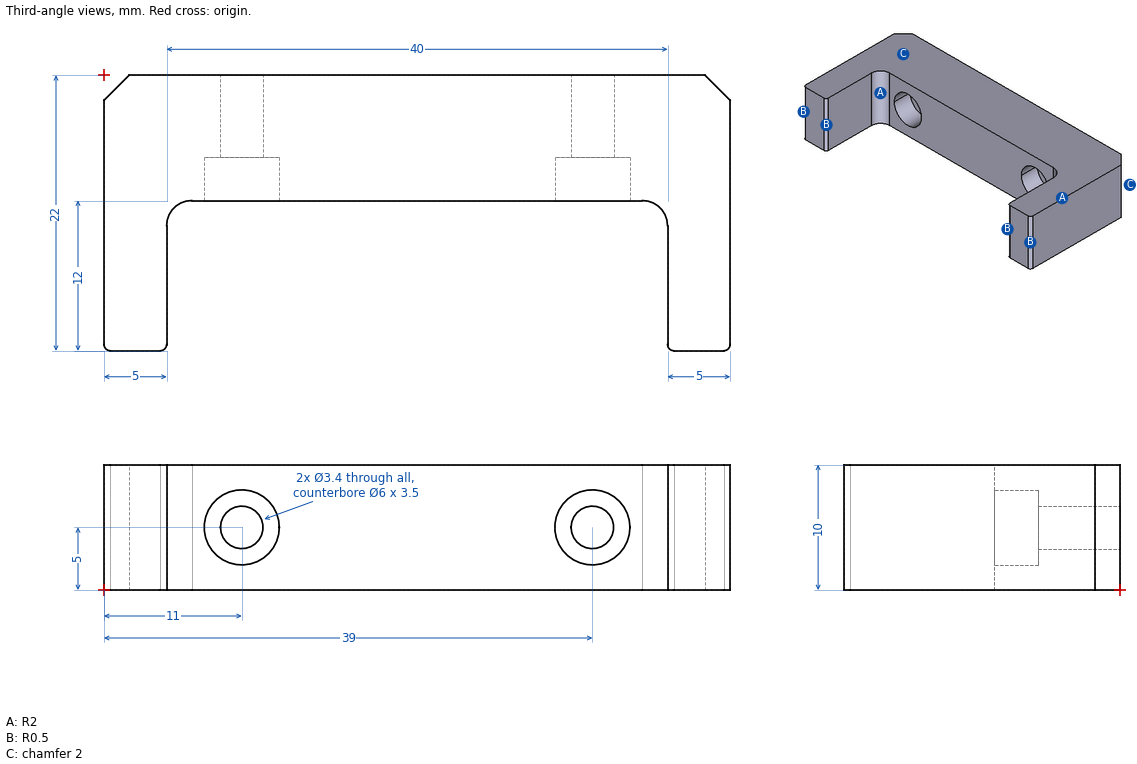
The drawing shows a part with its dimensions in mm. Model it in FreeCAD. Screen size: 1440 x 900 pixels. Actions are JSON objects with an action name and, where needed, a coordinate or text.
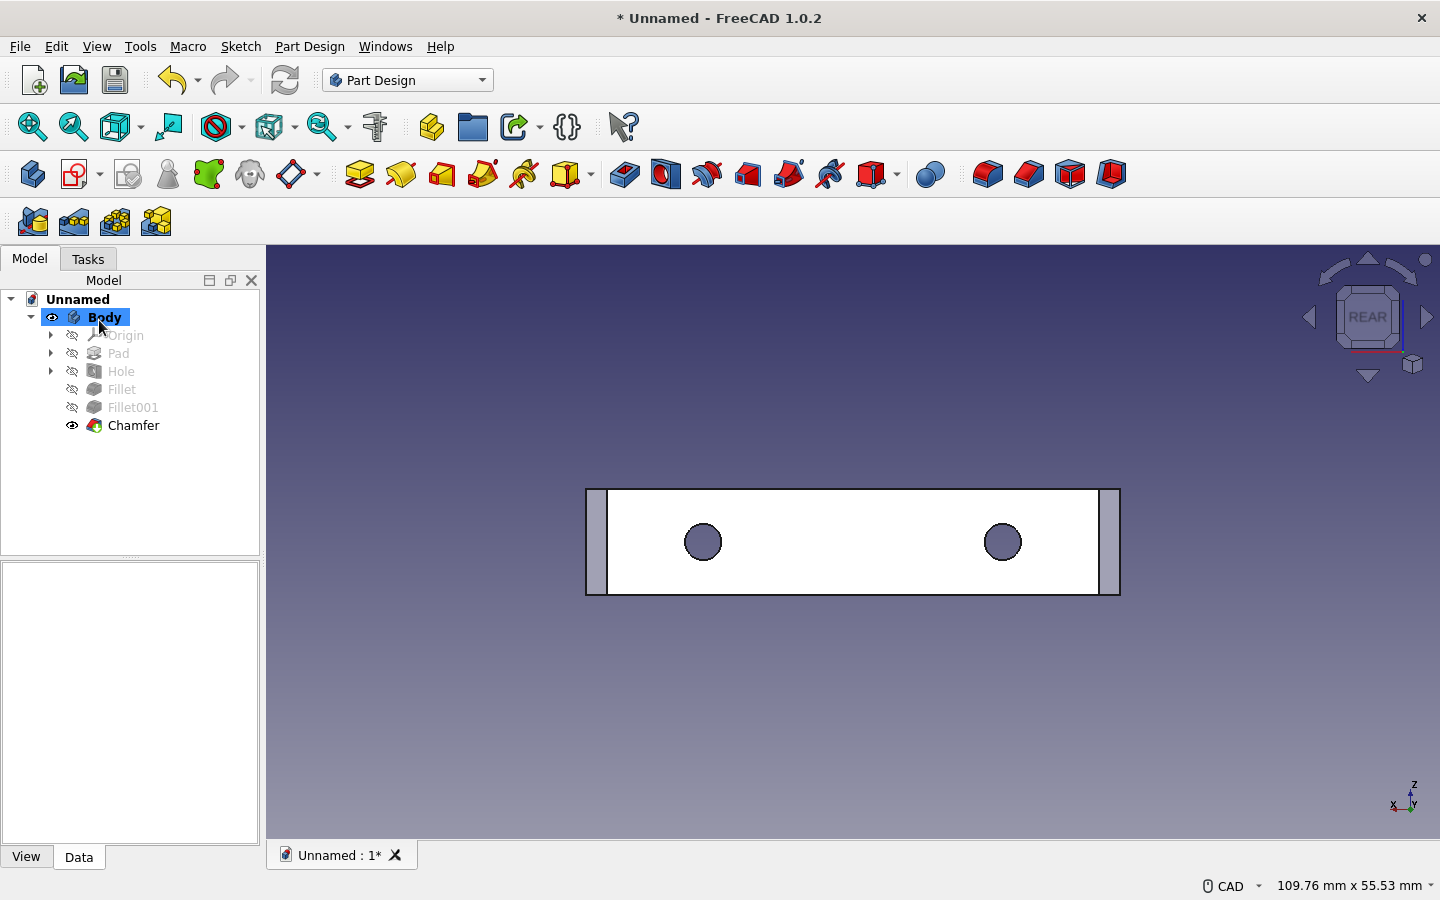
{"action": "key", "text": "0"}